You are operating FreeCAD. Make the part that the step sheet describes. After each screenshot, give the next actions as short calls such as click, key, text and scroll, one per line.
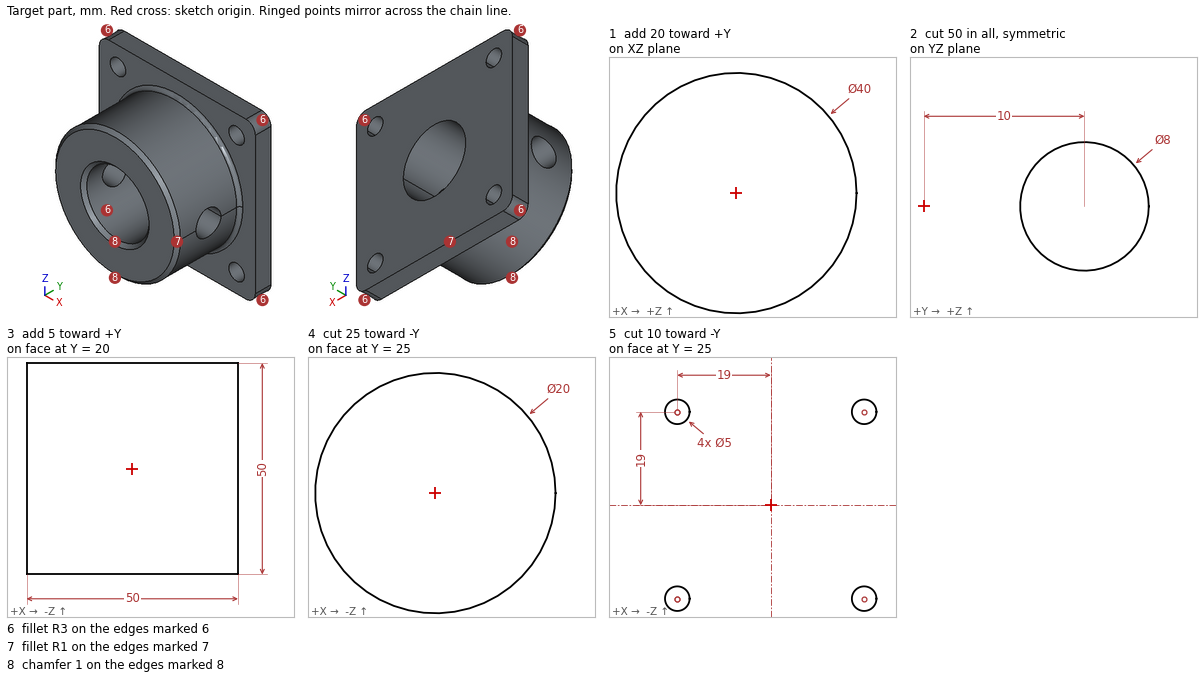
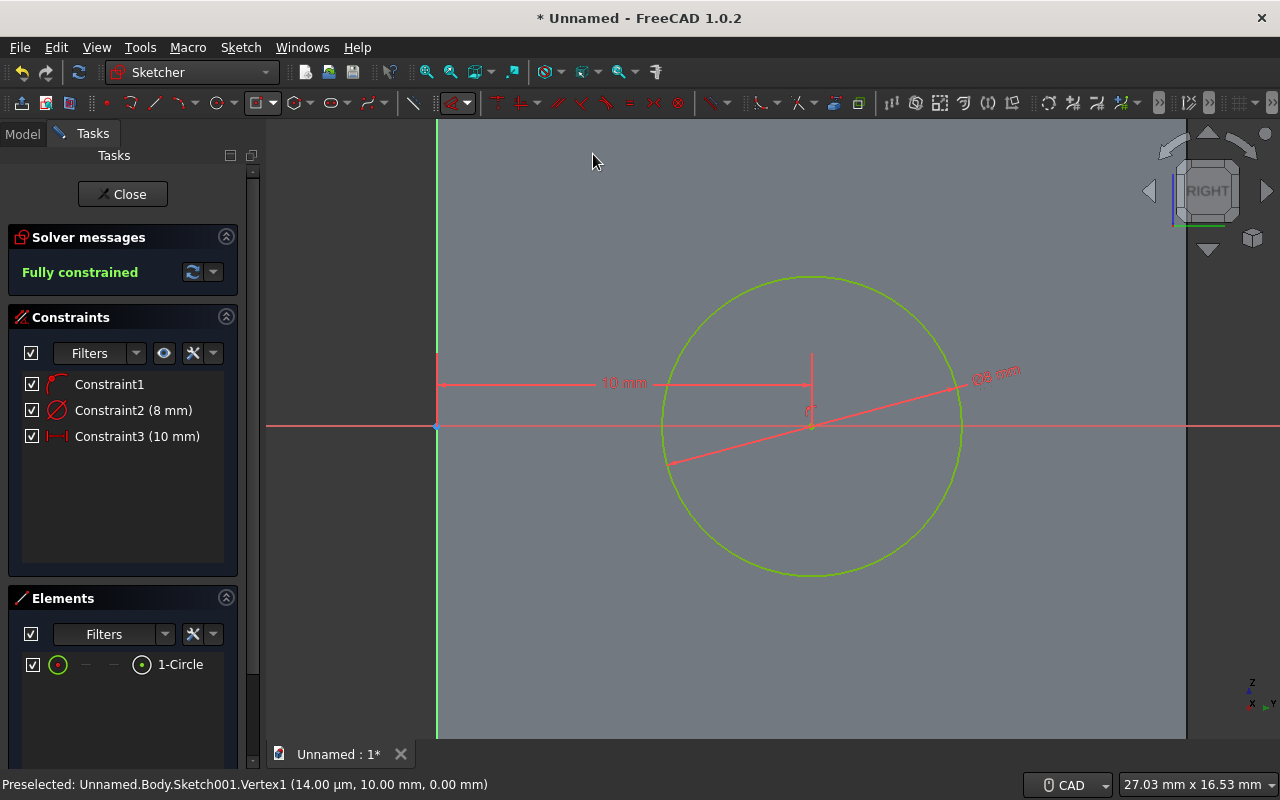
click(123, 194)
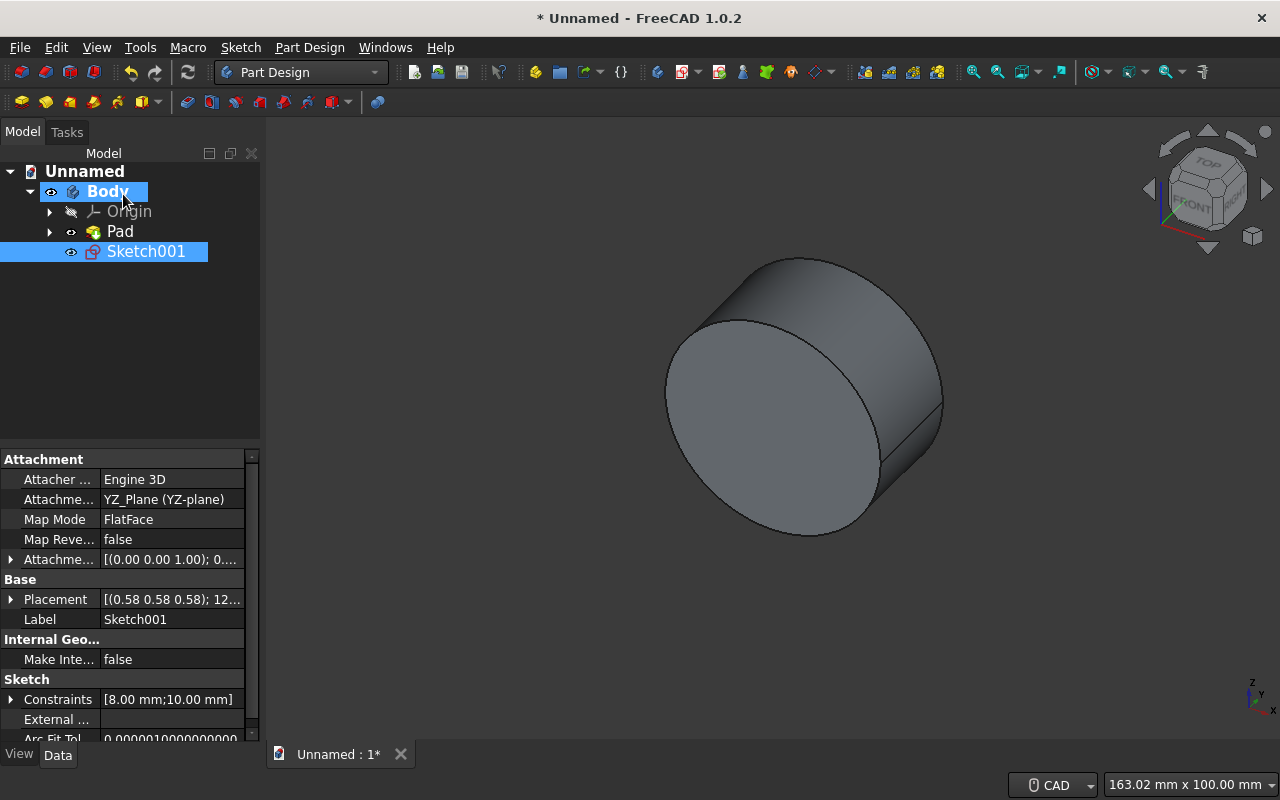
click(188, 102)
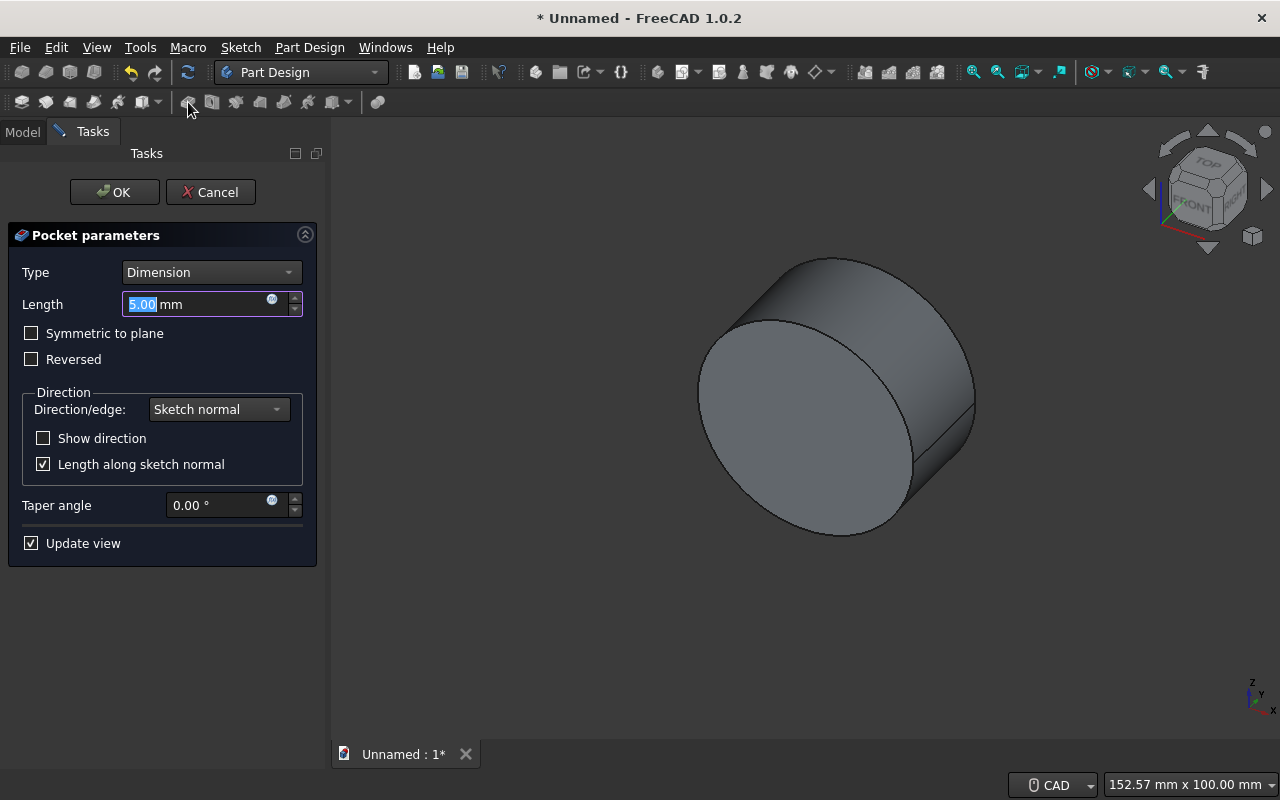
text(50)
key(Tab)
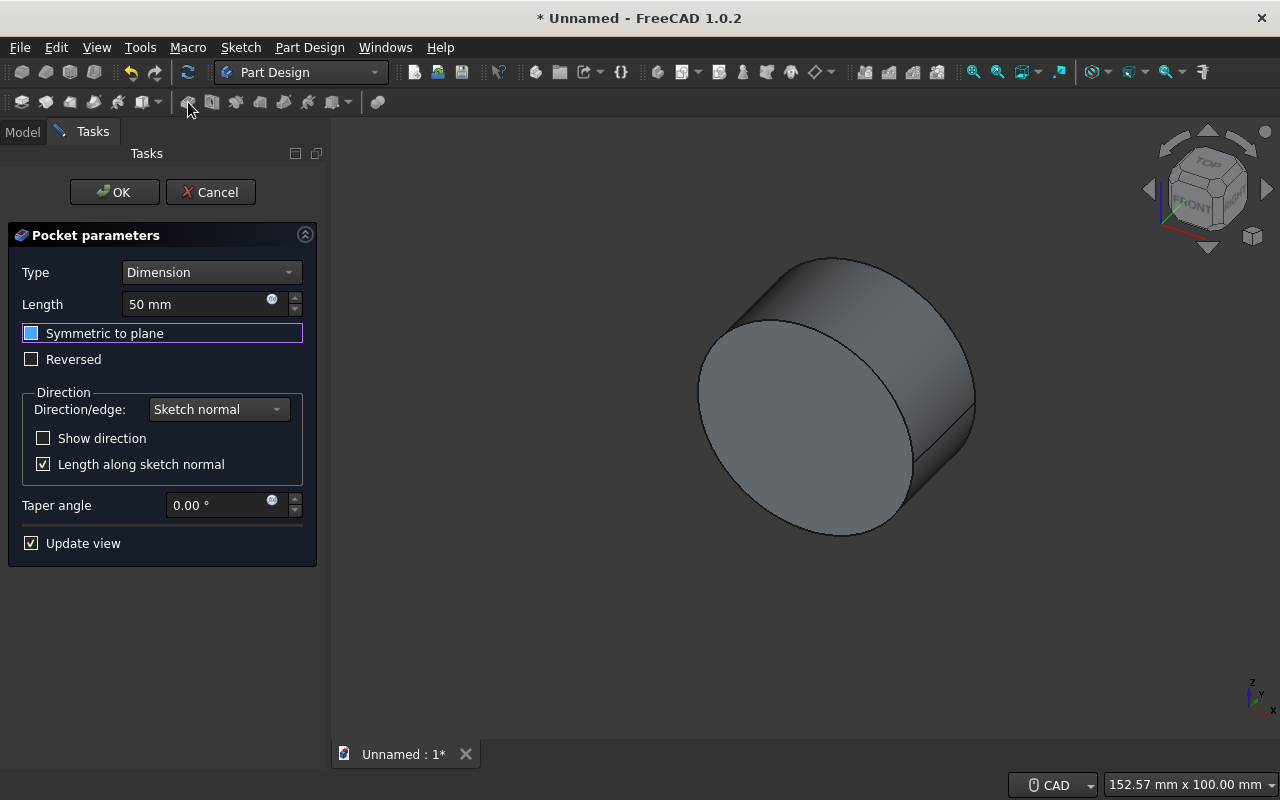
click(30, 333)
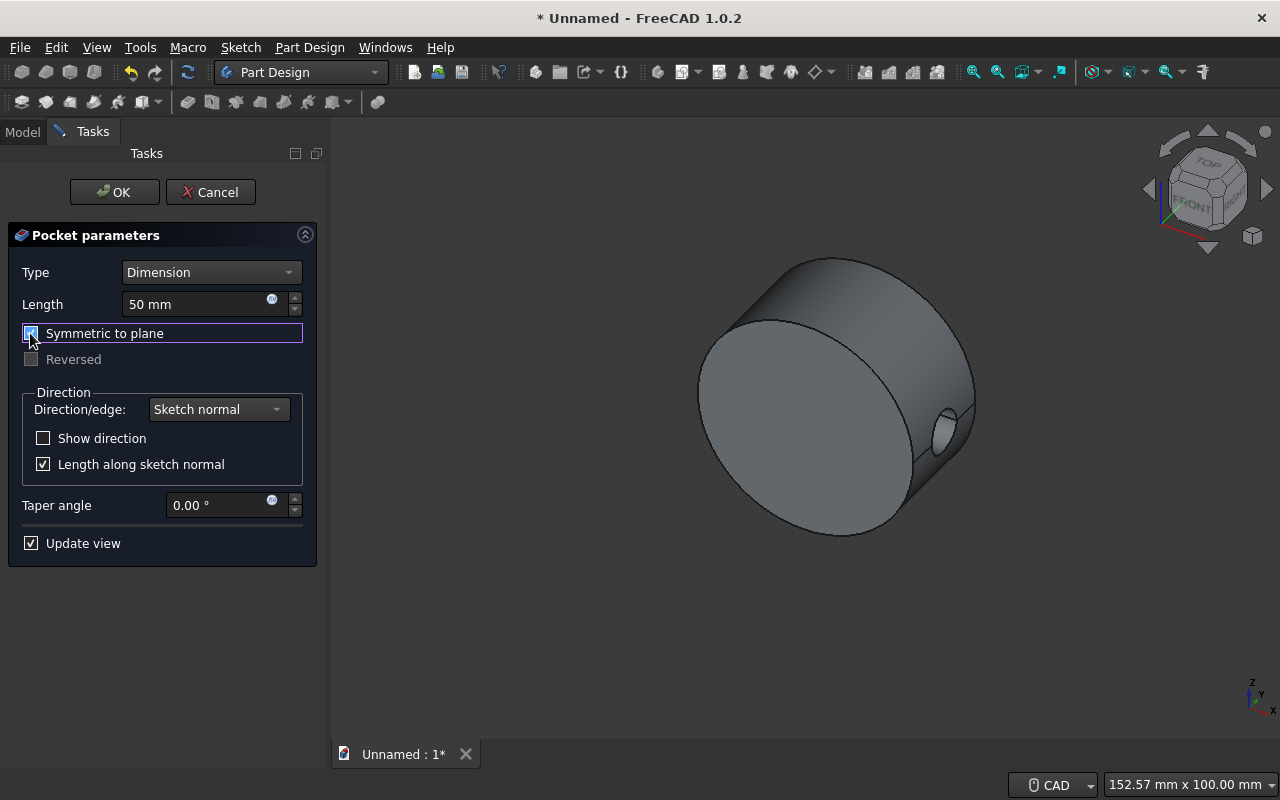
click(115, 192)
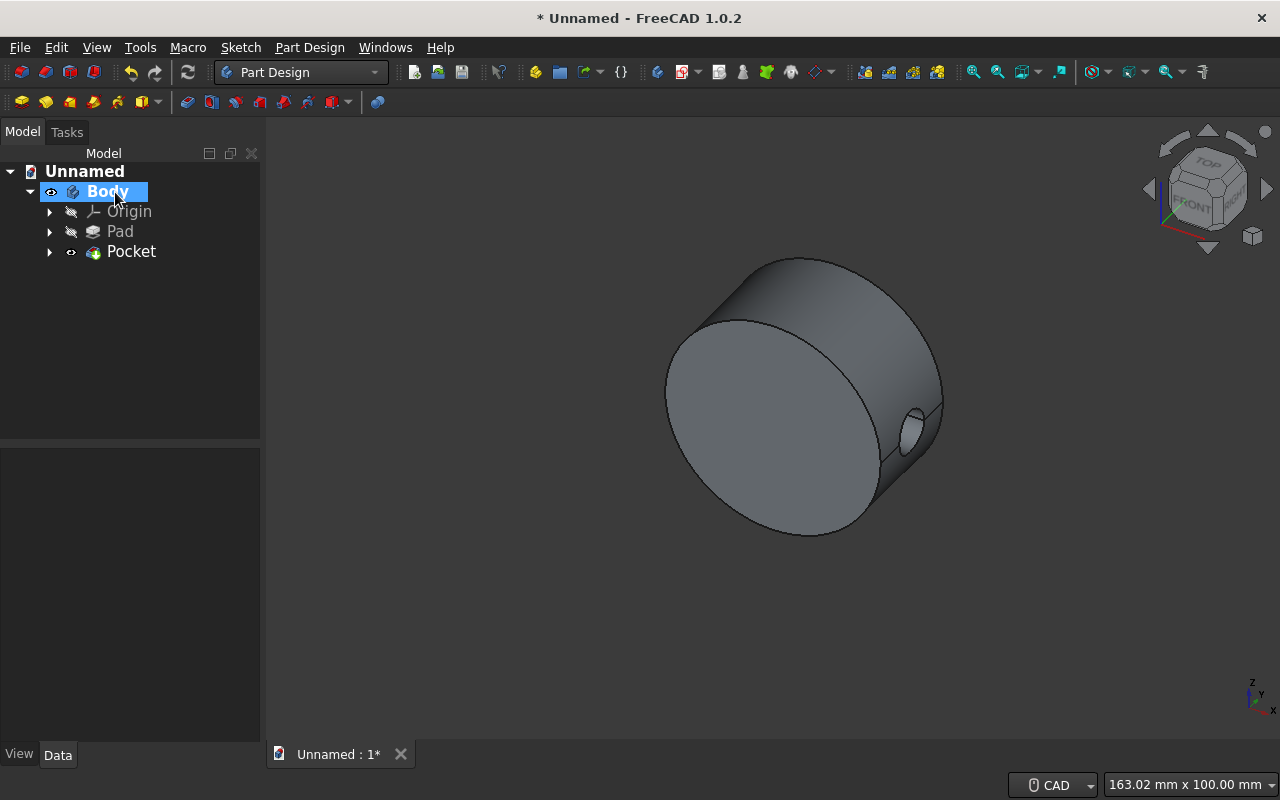
key(4)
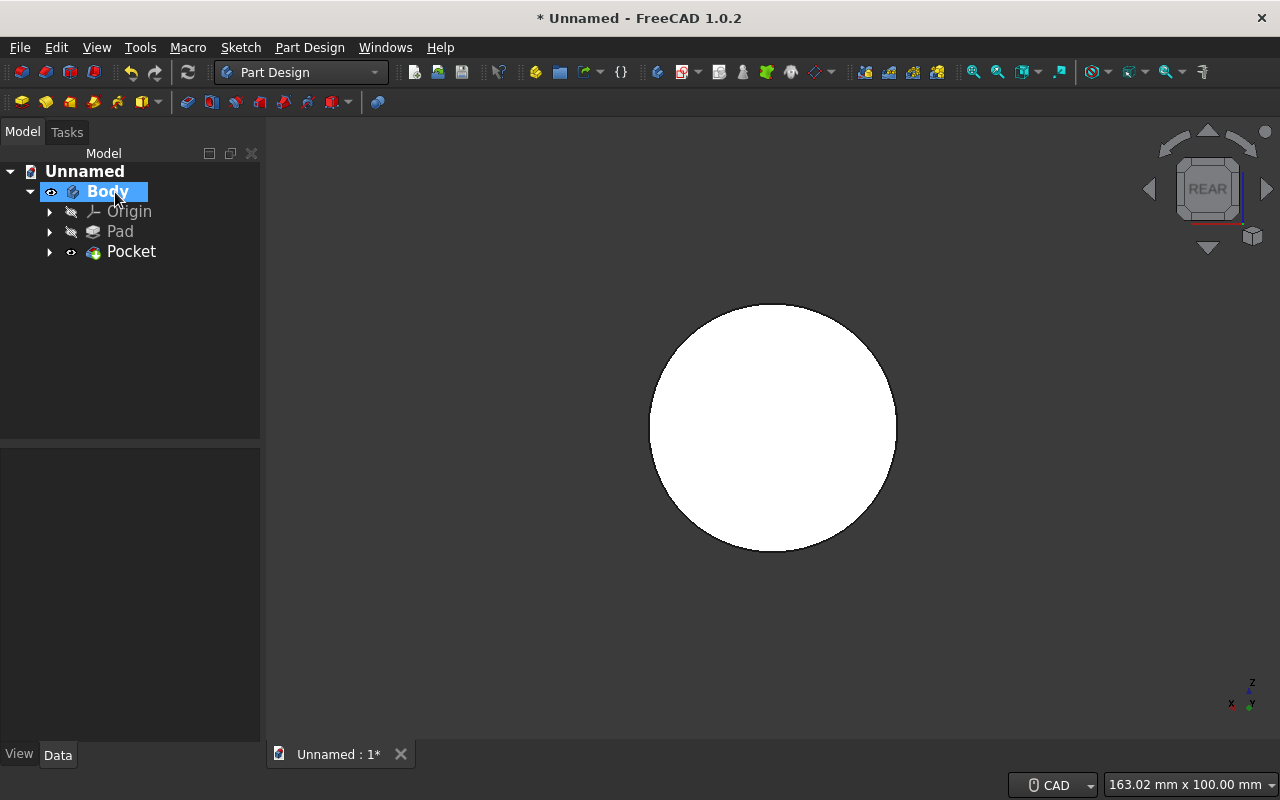
click(974, 72)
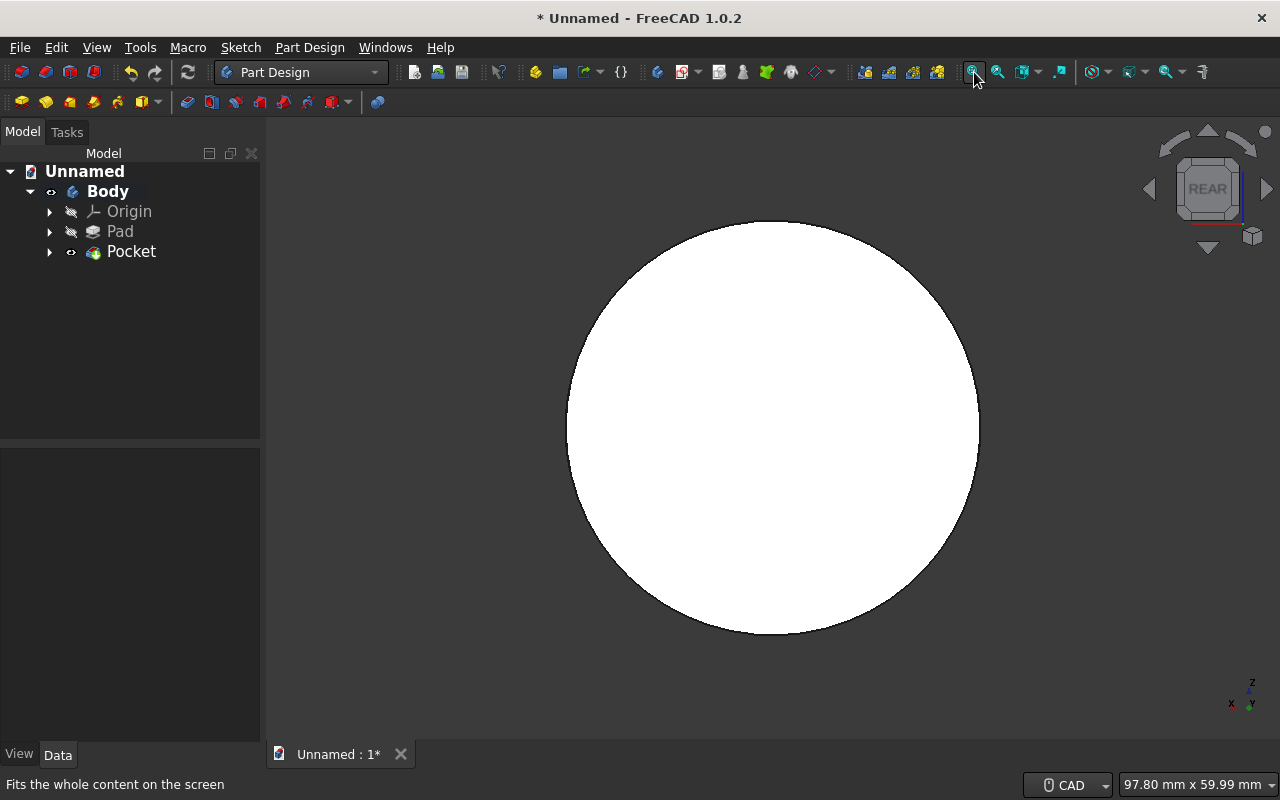
click(773, 427)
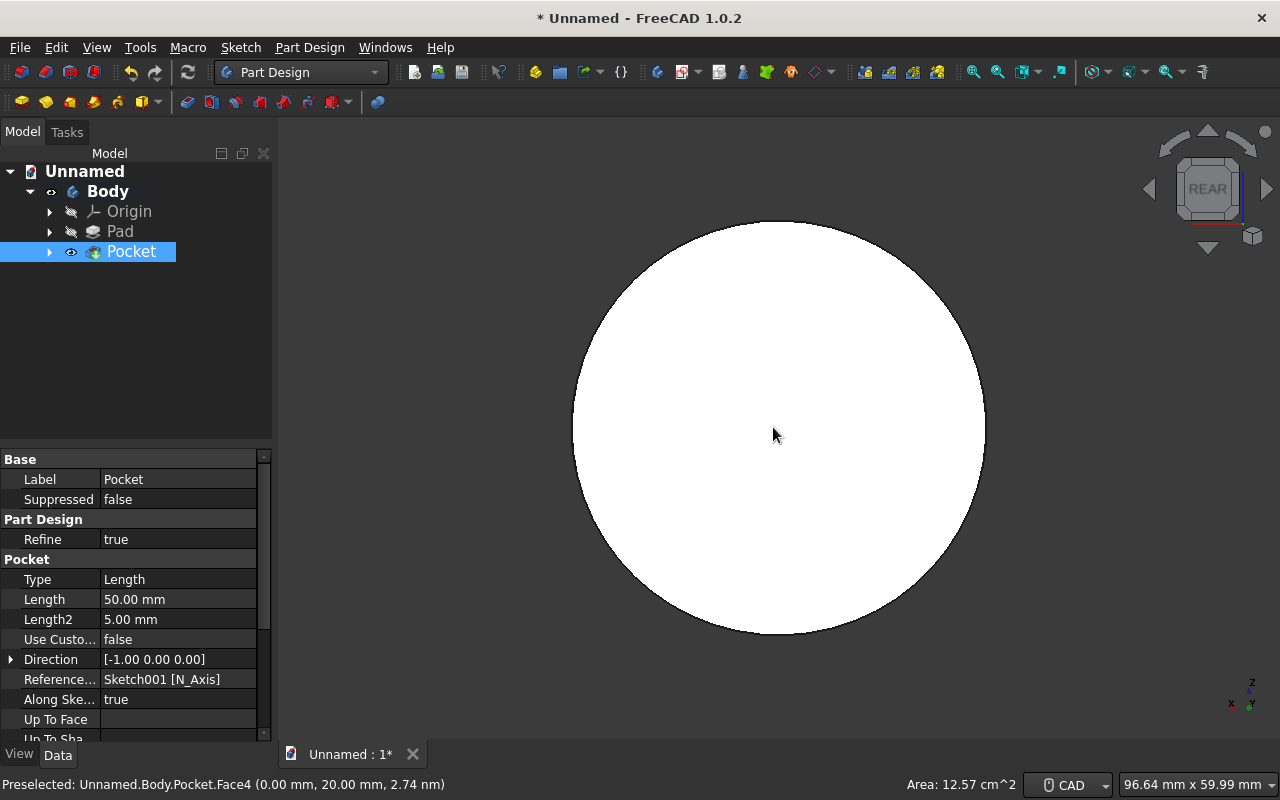
click(682, 72)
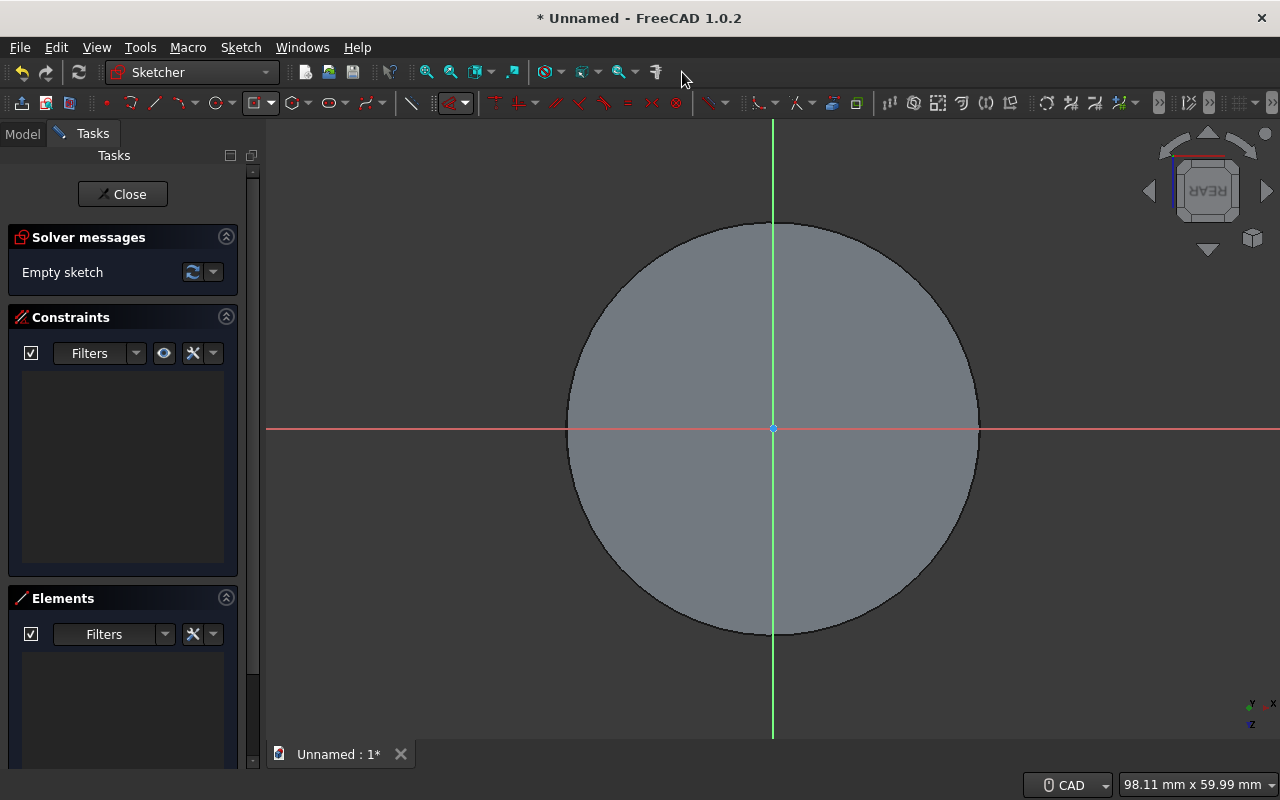
scroll(395, 429, down, 1)